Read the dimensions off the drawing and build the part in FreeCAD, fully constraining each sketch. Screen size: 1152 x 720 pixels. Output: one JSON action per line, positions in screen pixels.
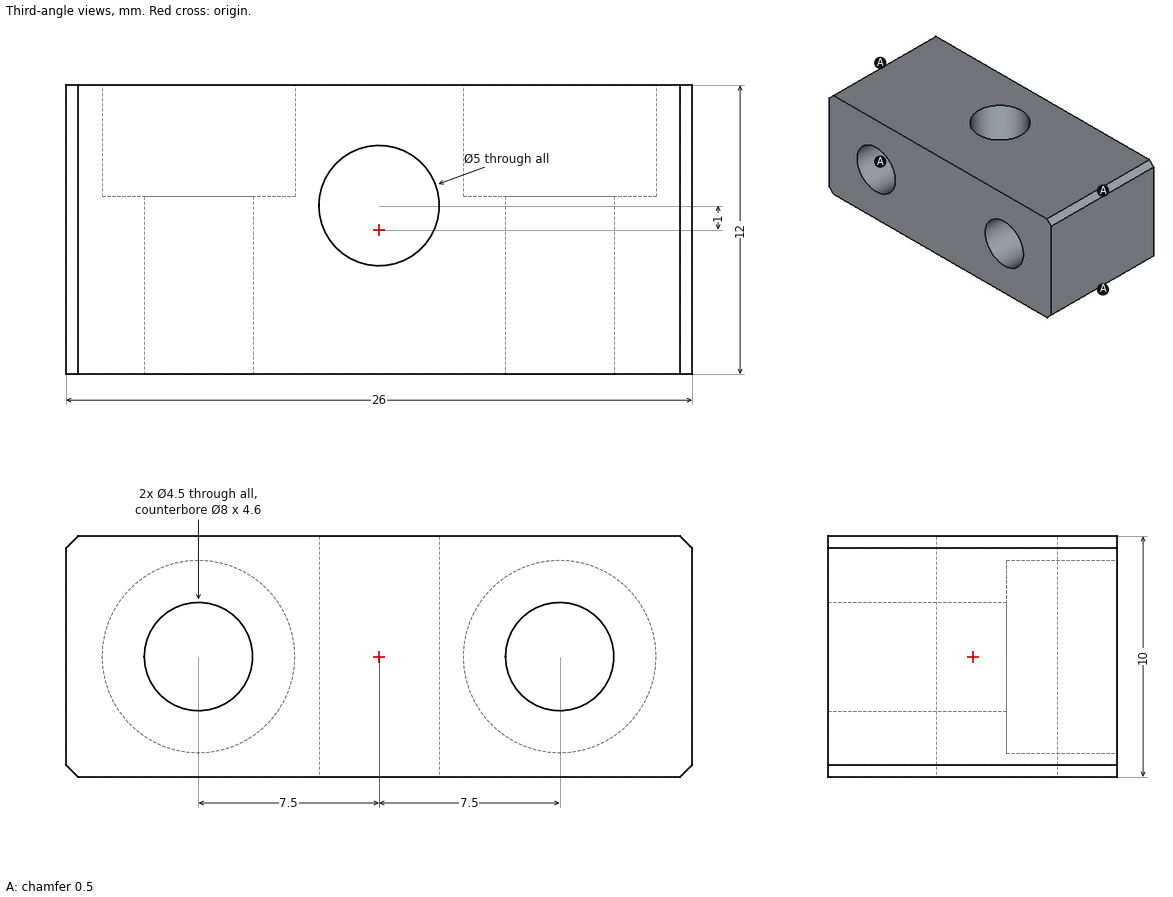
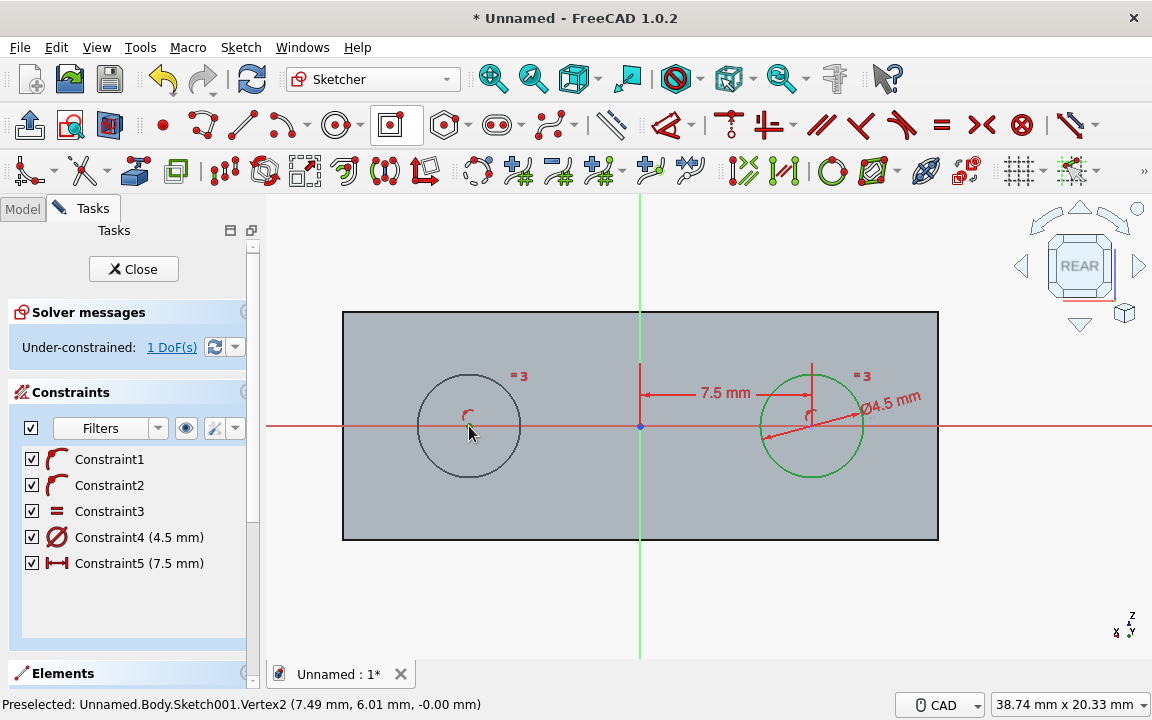
{"action": "key", "text": "l"}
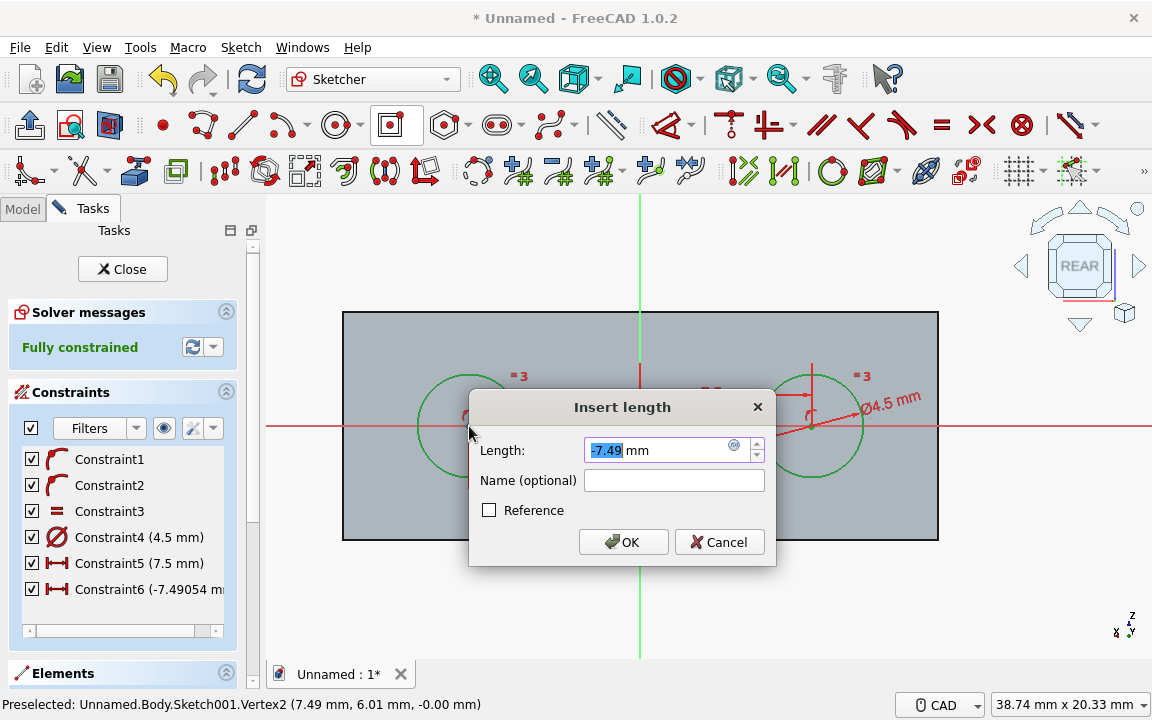
{"action": "type", "text": "-7.5"}
{"action": "key", "text": "Return"}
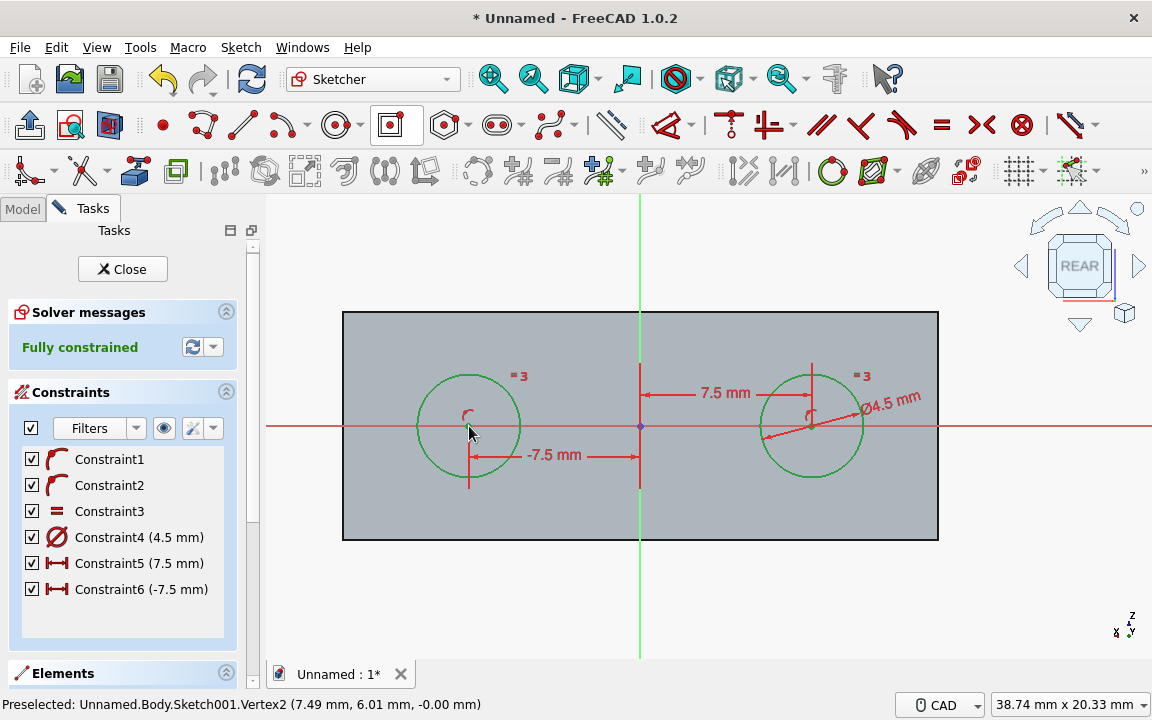
{"action": "left_click", "coordinate": [123, 269]}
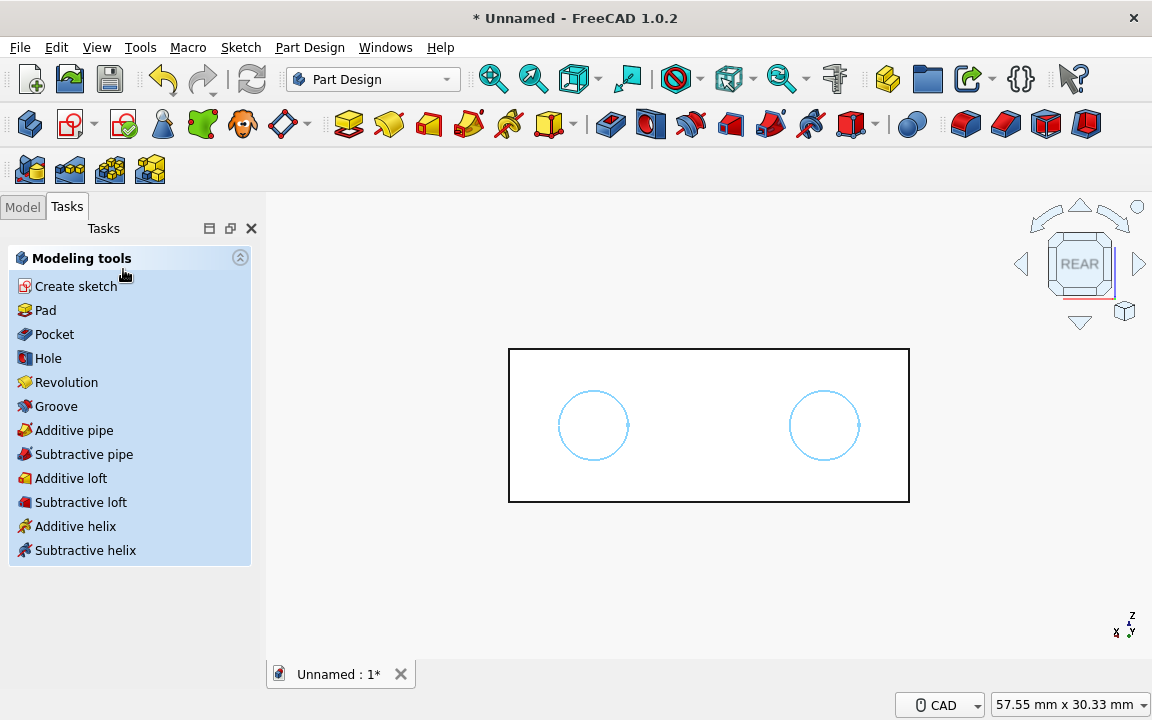
{"action": "left_click", "coordinate": [652, 124]}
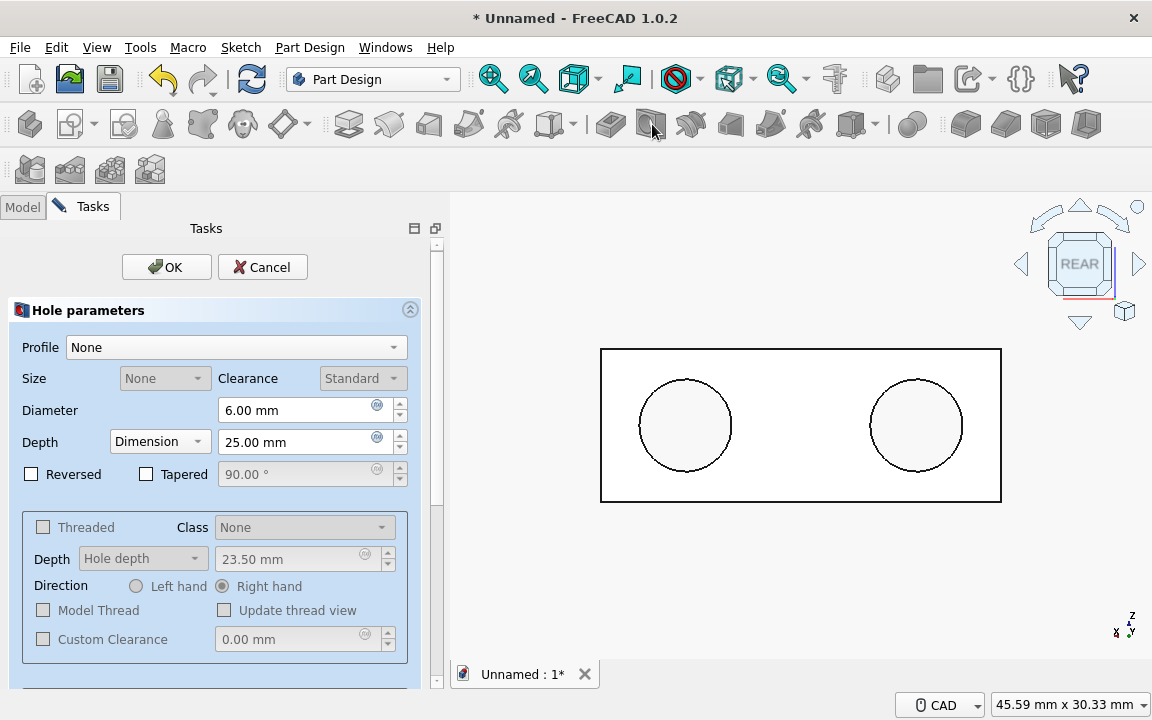
{"action": "triple_click", "coordinate": [305, 410]}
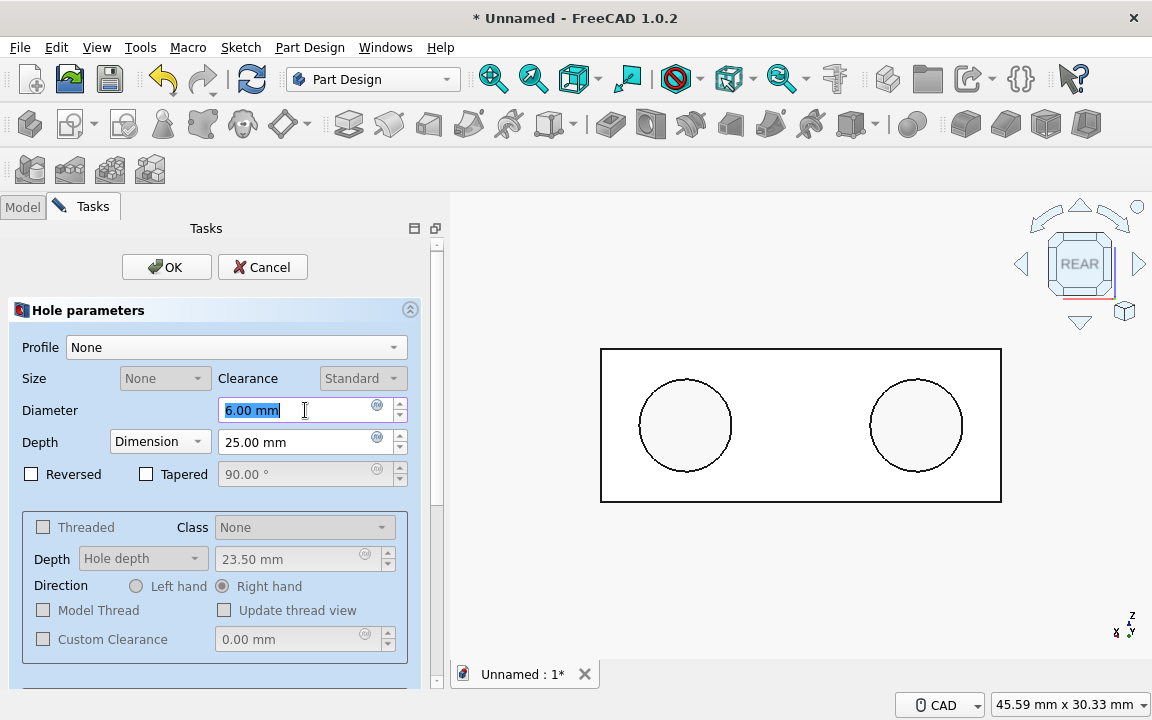
{"action": "type", "text": "4.5"}
{"action": "key", "text": "Tab"}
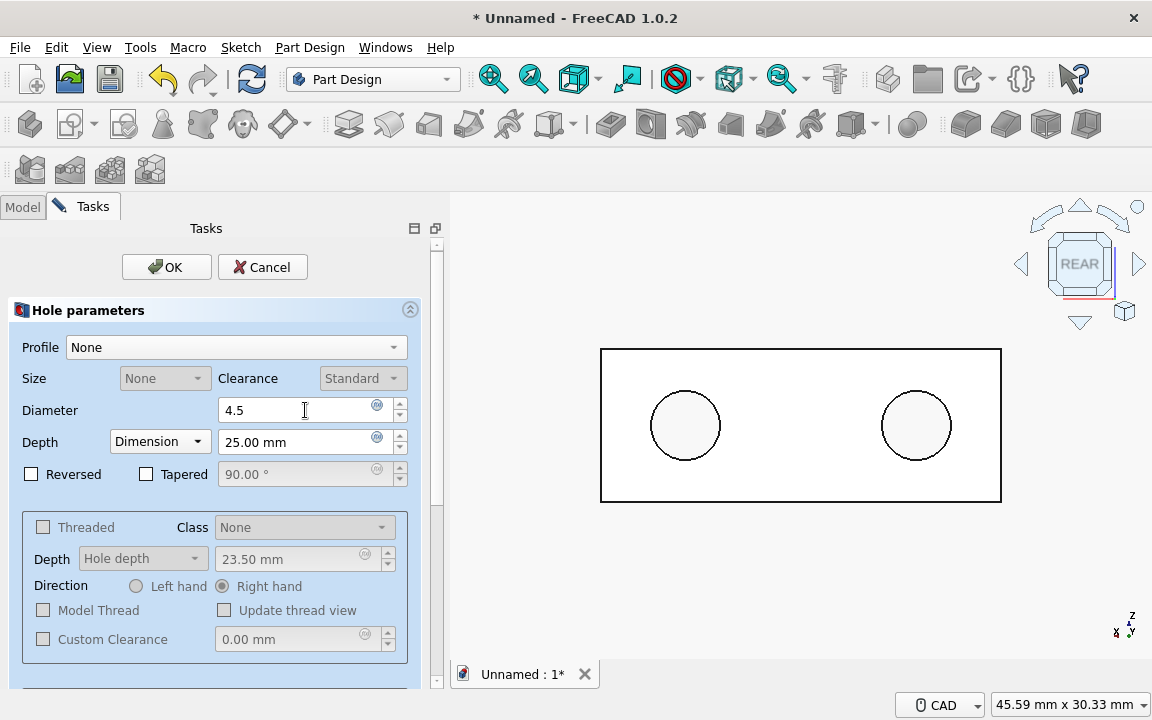
{"action": "left_click", "coordinate": [161, 442]}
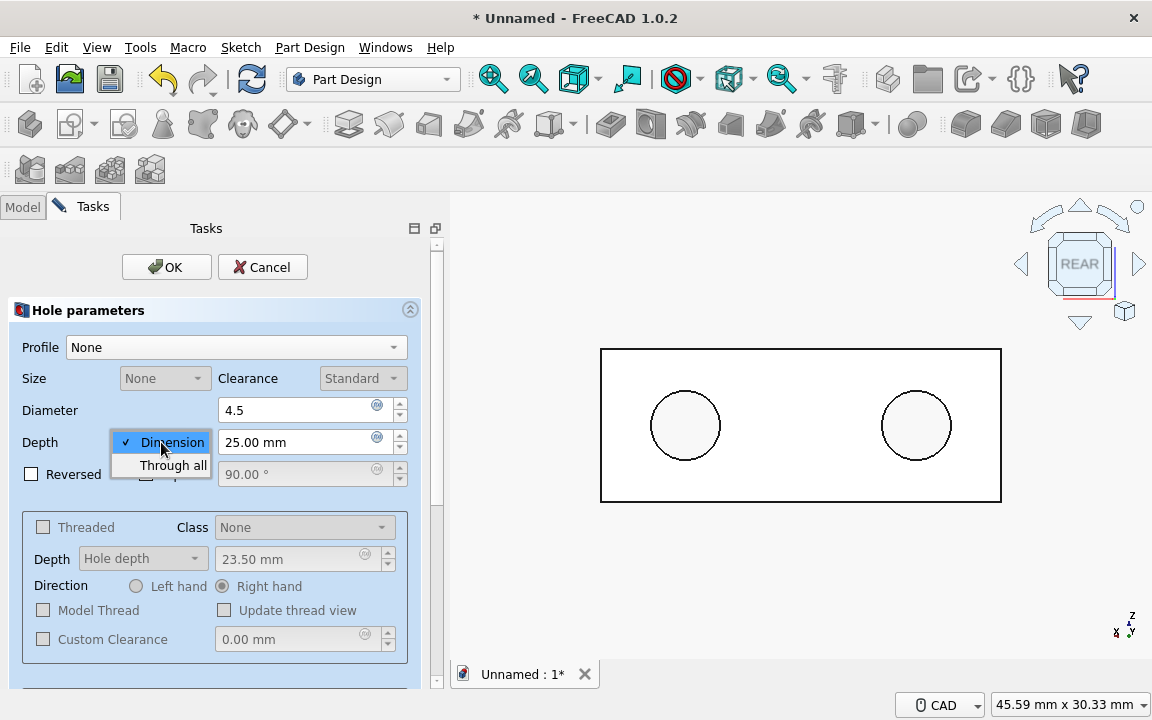
{"action": "left_click", "coordinate": [160, 466]}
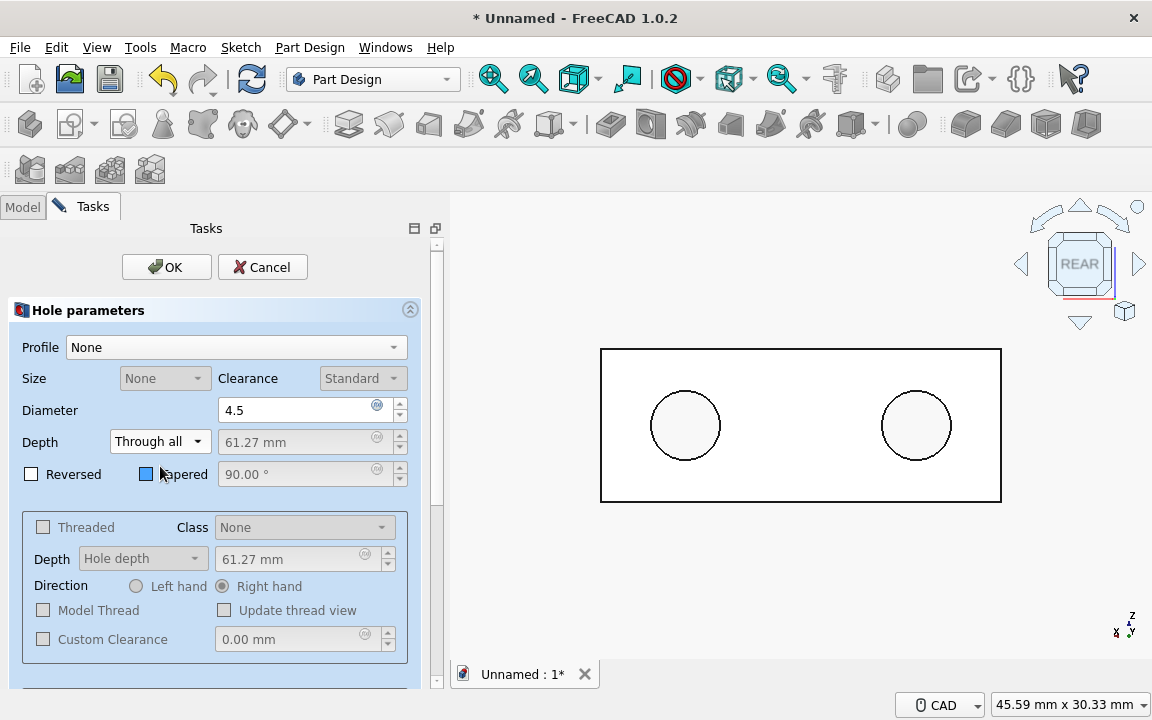
{"action": "scroll", "coordinate": [437, 463], "scroll_direction": "down", "scroll_amount": 2}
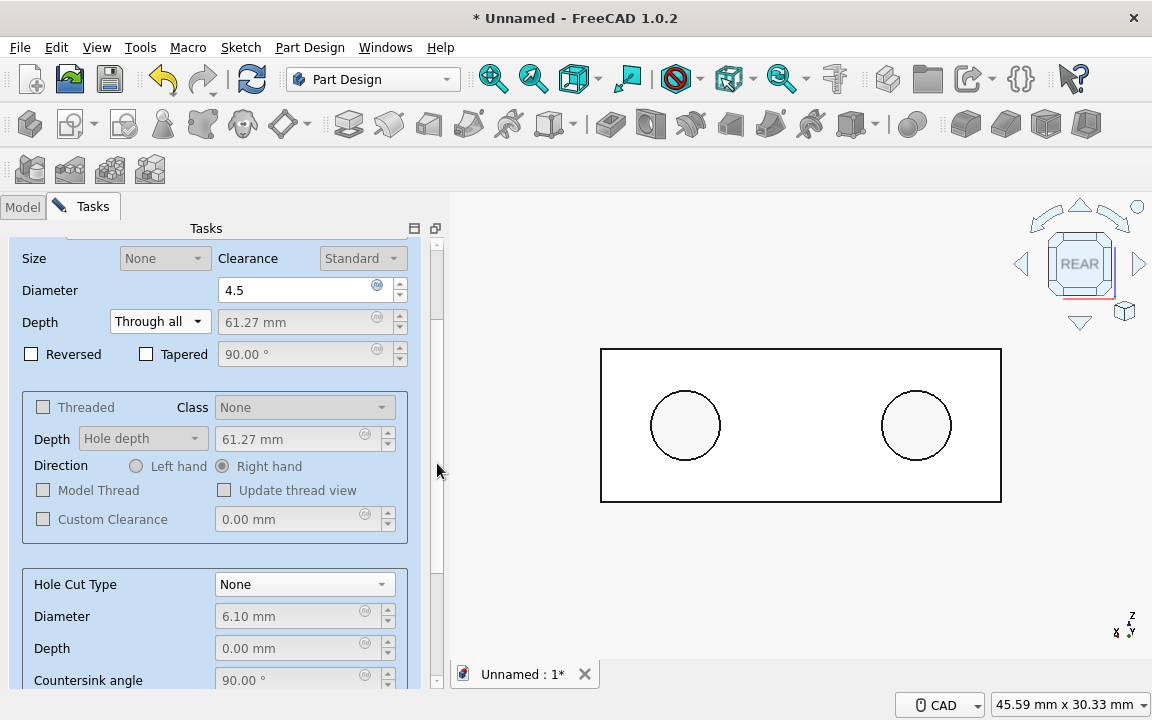
{"action": "left_click", "coordinate": [306, 584]}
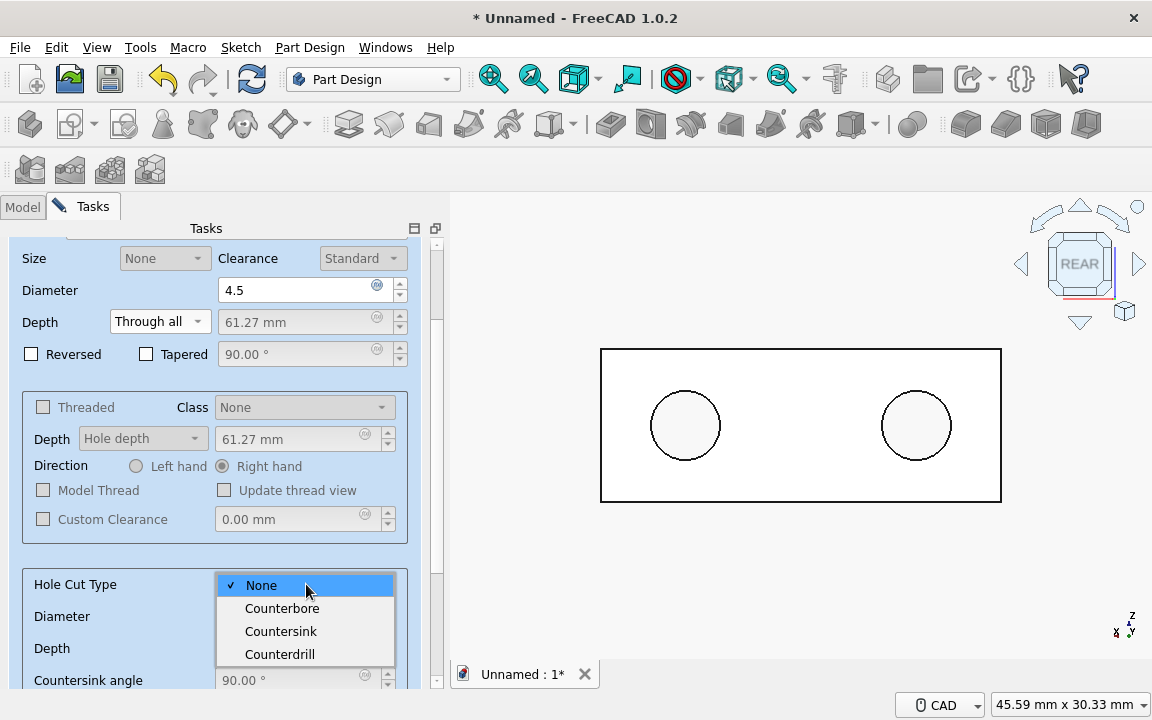
{"action": "left_click", "coordinate": [304, 608]}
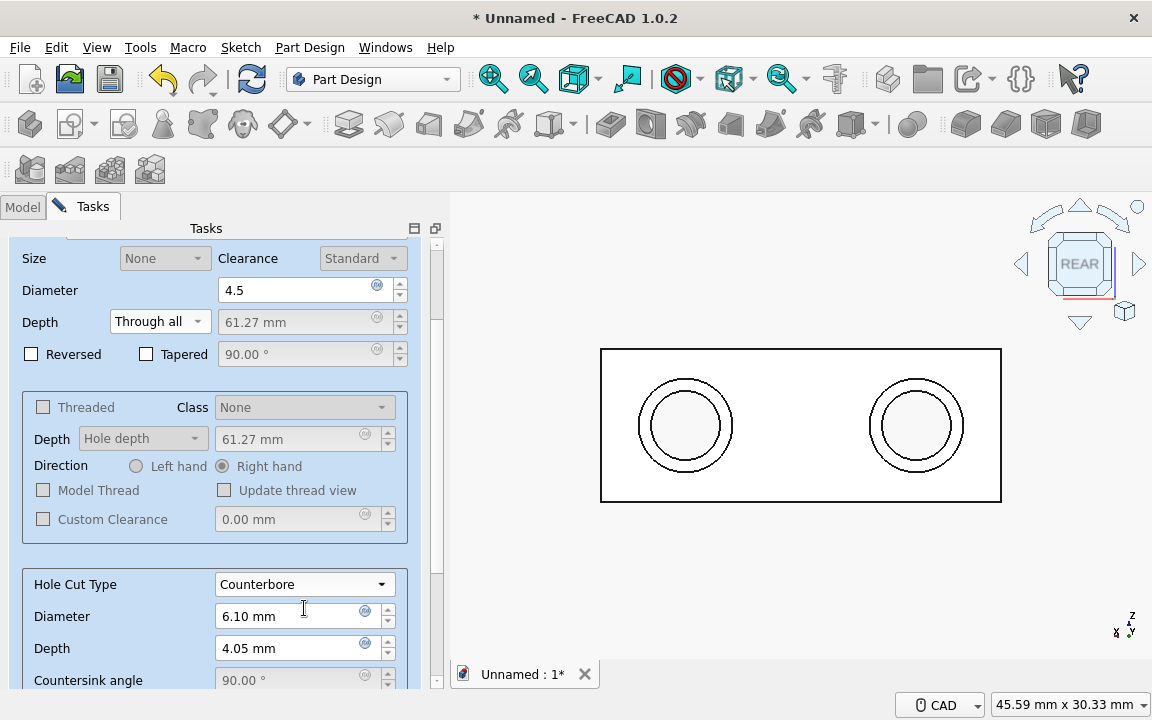
{"action": "triple_click", "coordinate": [298, 616]}